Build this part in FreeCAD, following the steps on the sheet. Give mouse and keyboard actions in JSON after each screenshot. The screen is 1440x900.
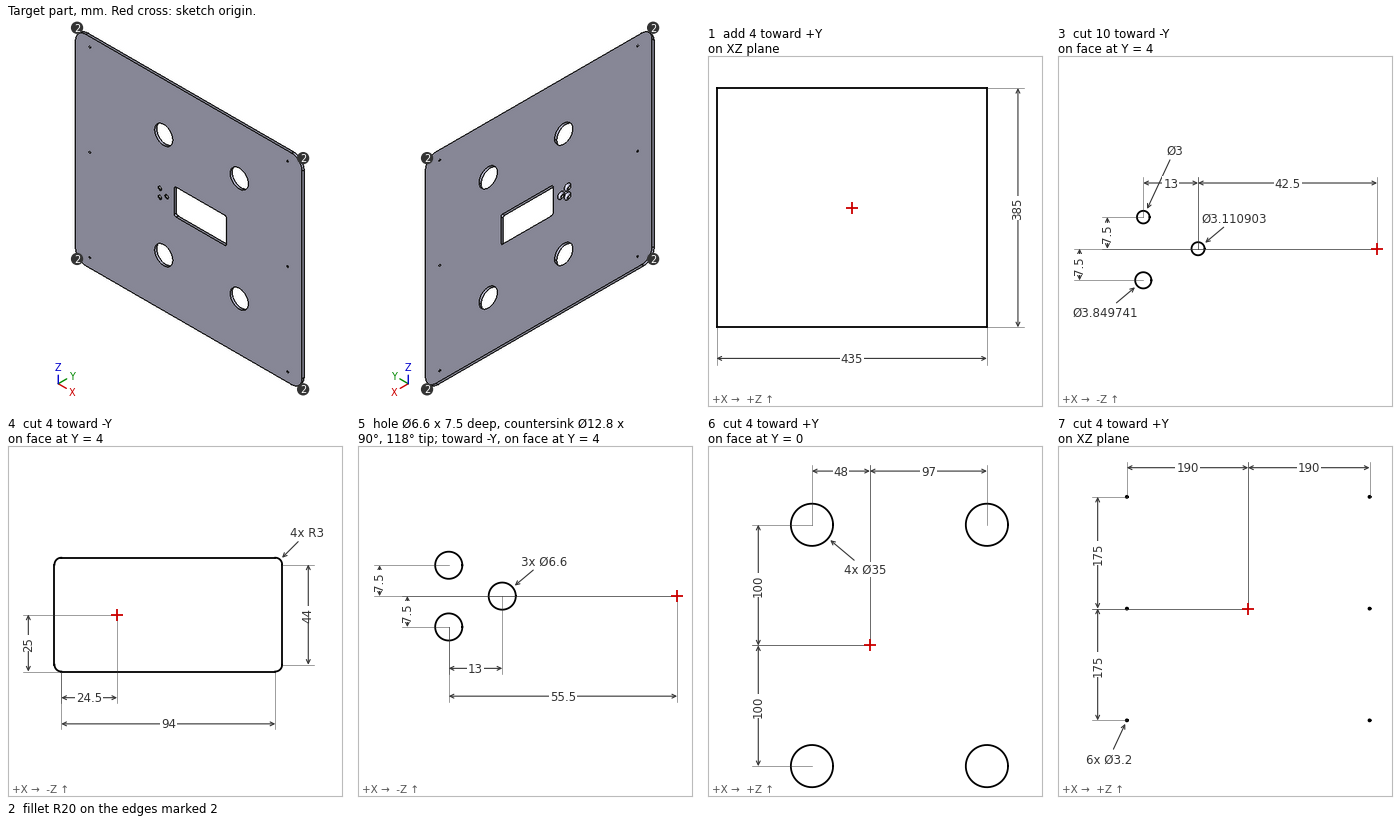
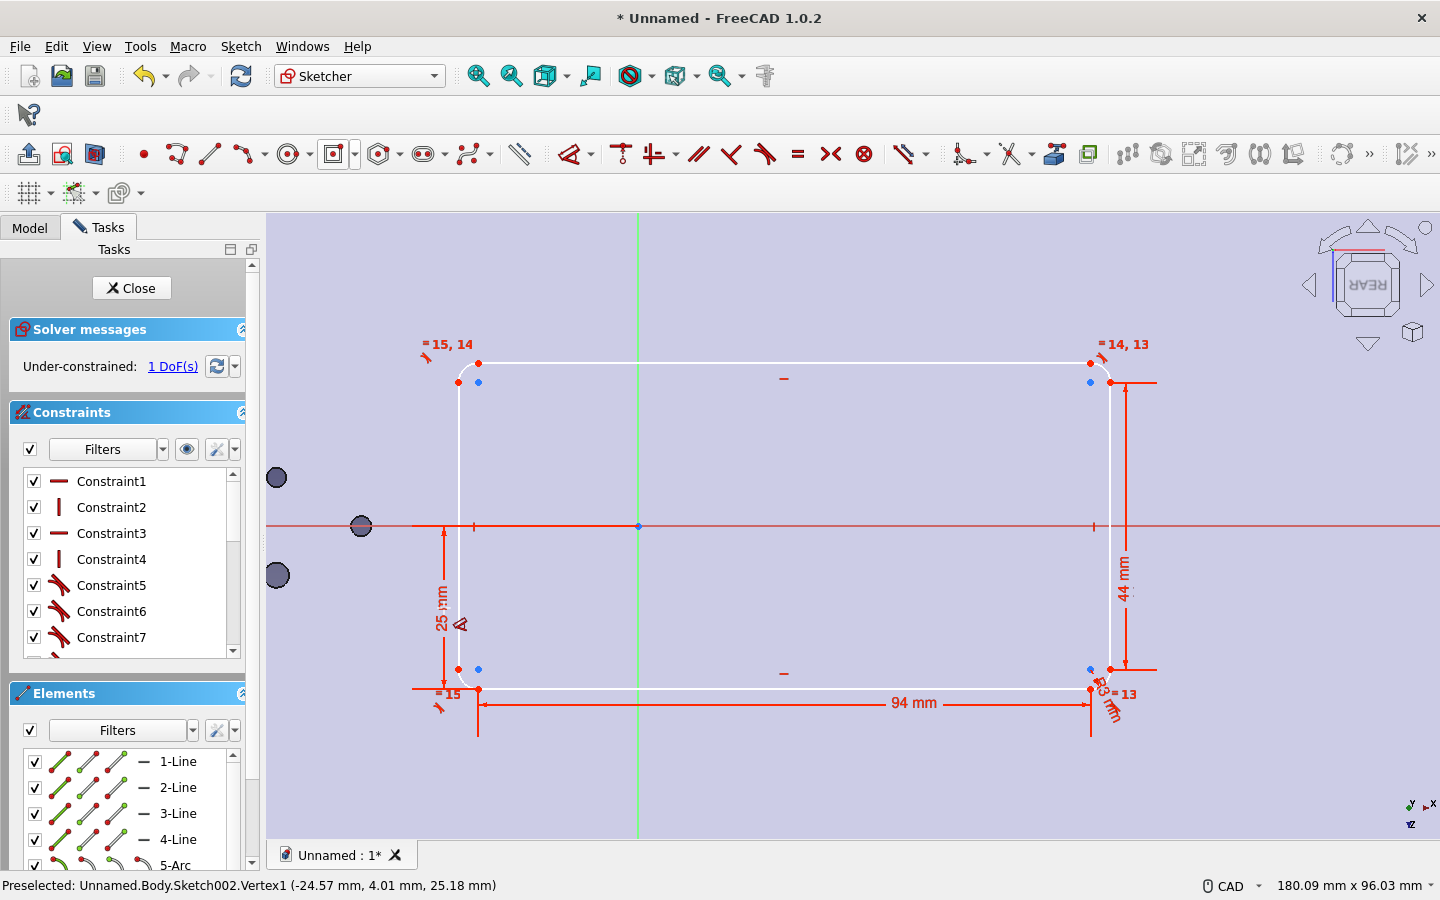
{"action": "left_click", "coordinate": [478, 689]}
{"action": "left_click", "coordinate": [558, 723]}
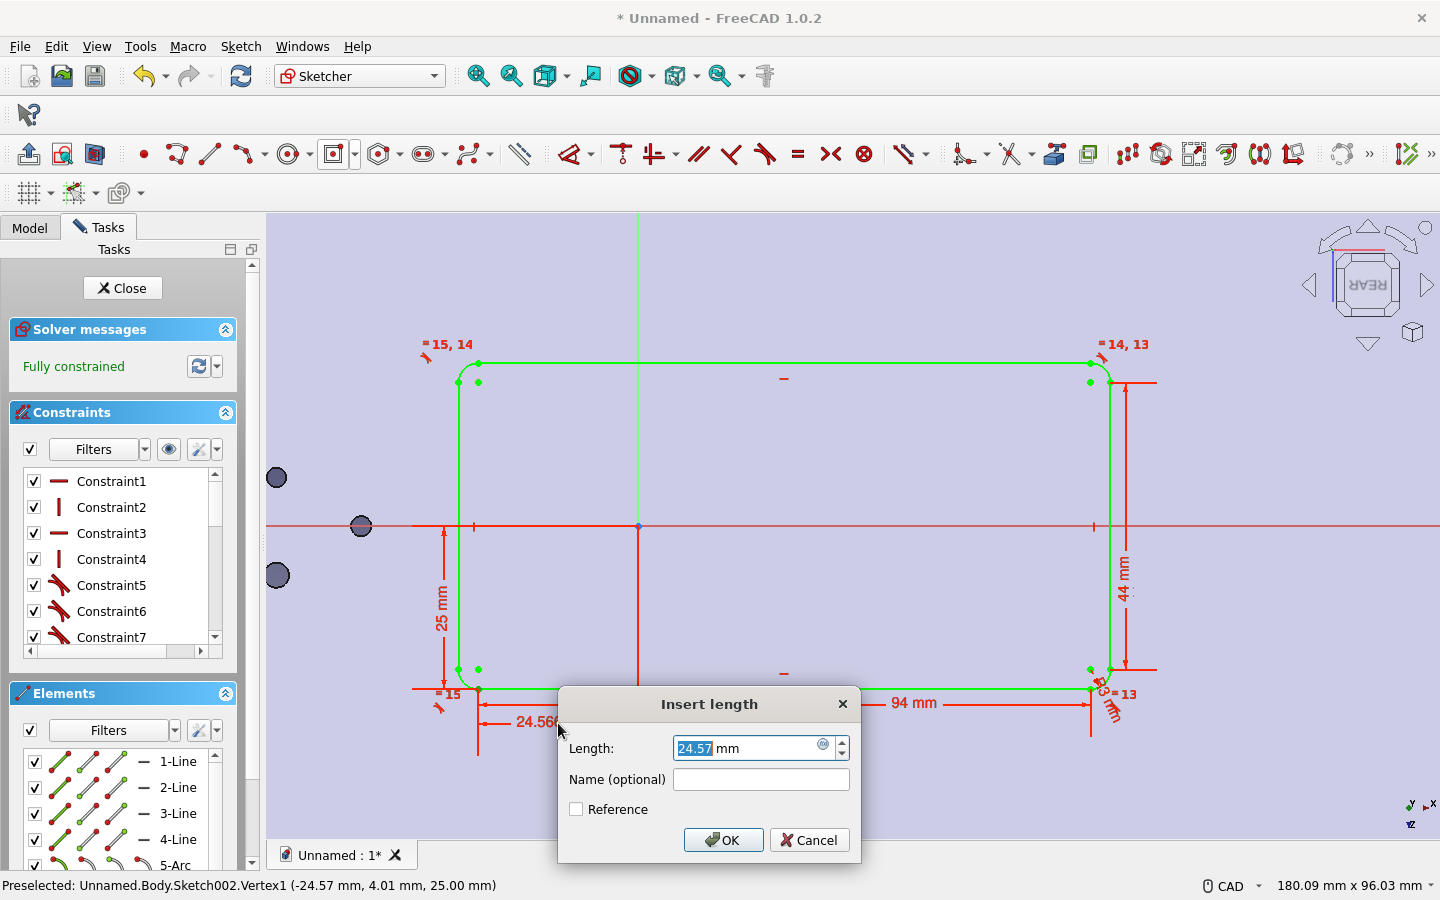
{"action": "type", "text": "24.5"}
{"action": "key", "text": "Return"}
{"action": "key", "text": "Escape"}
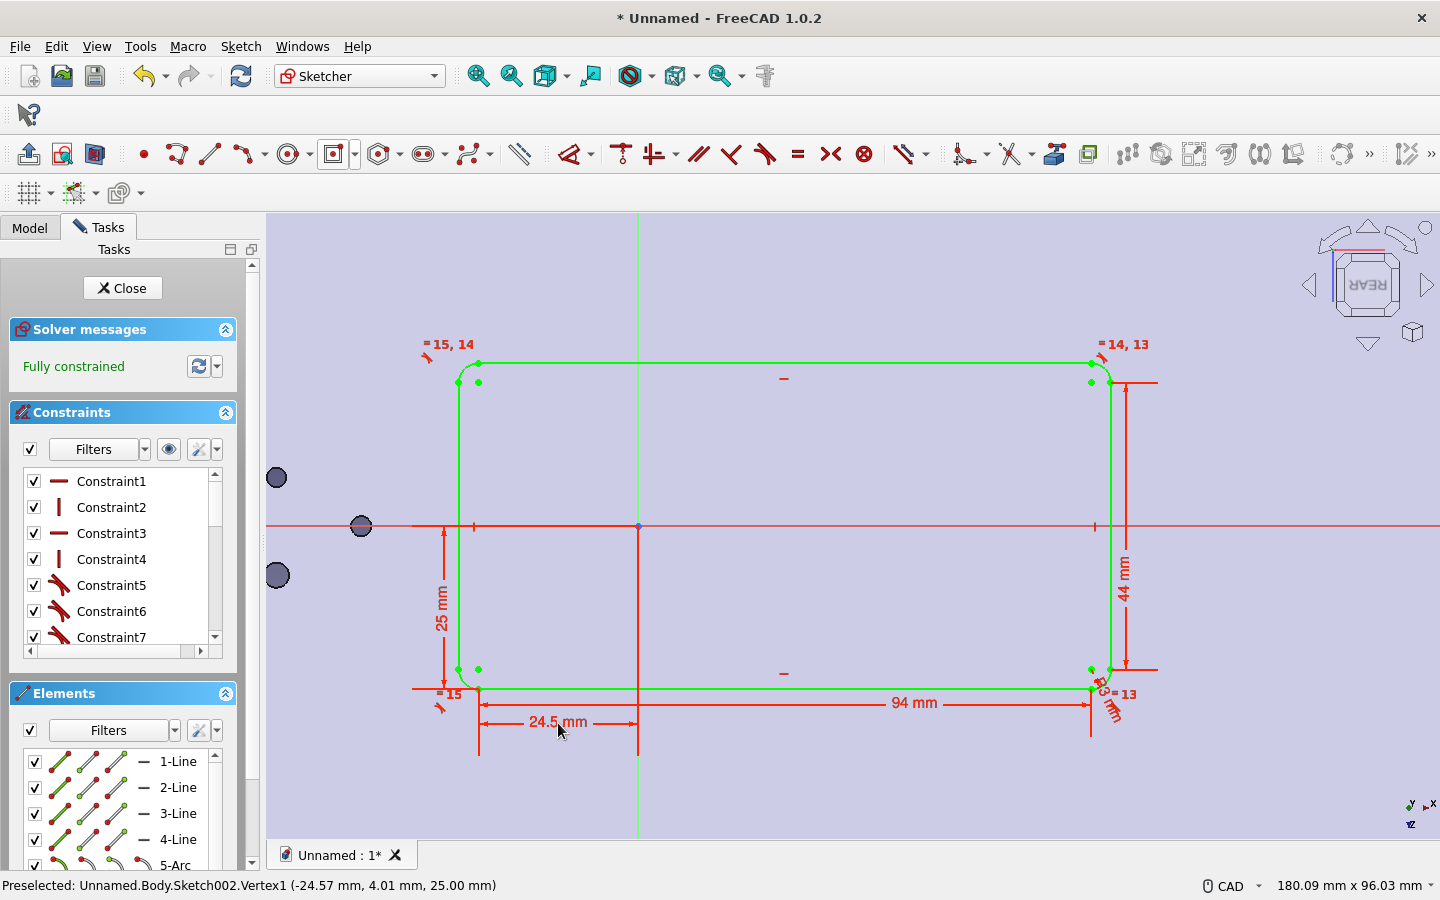
{"action": "left_click", "coordinate": [123, 288]}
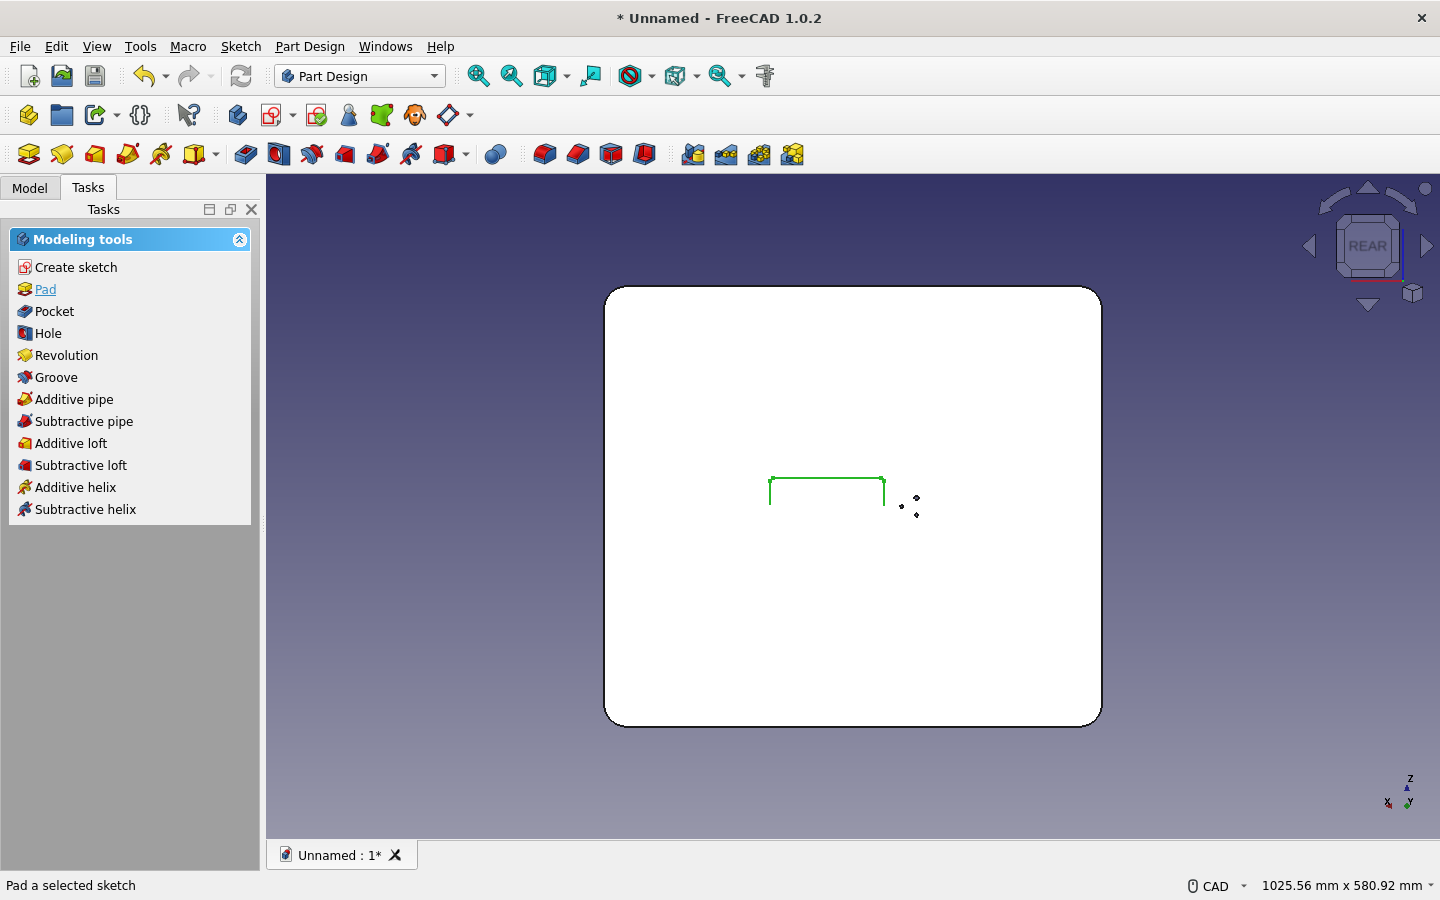
{"action": "left_click", "coordinate": [246, 154]}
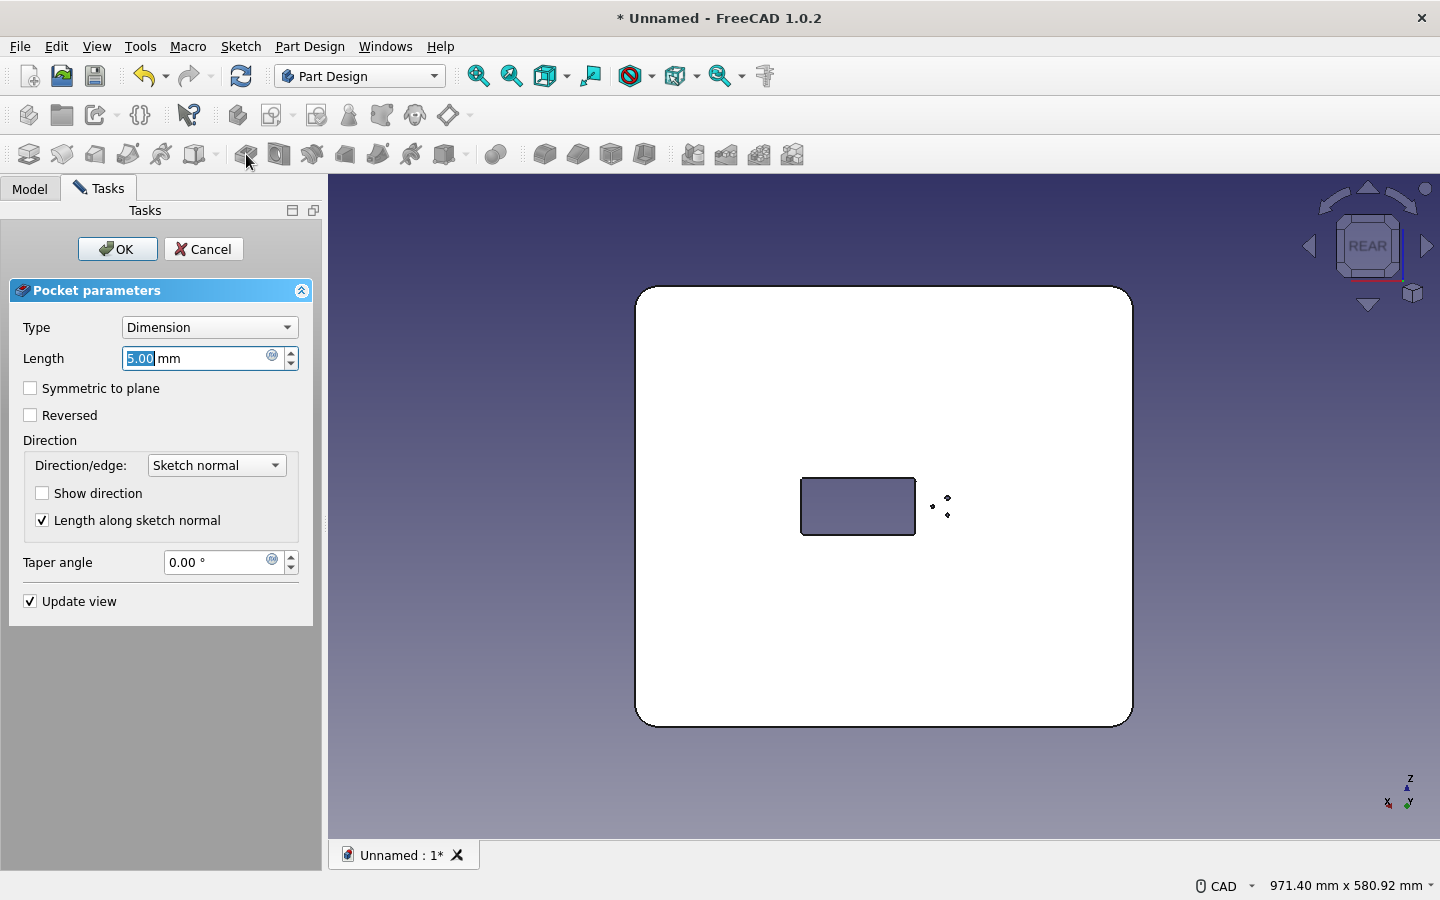
{"action": "type", "text": "4"}
{"action": "key", "text": "Tab"}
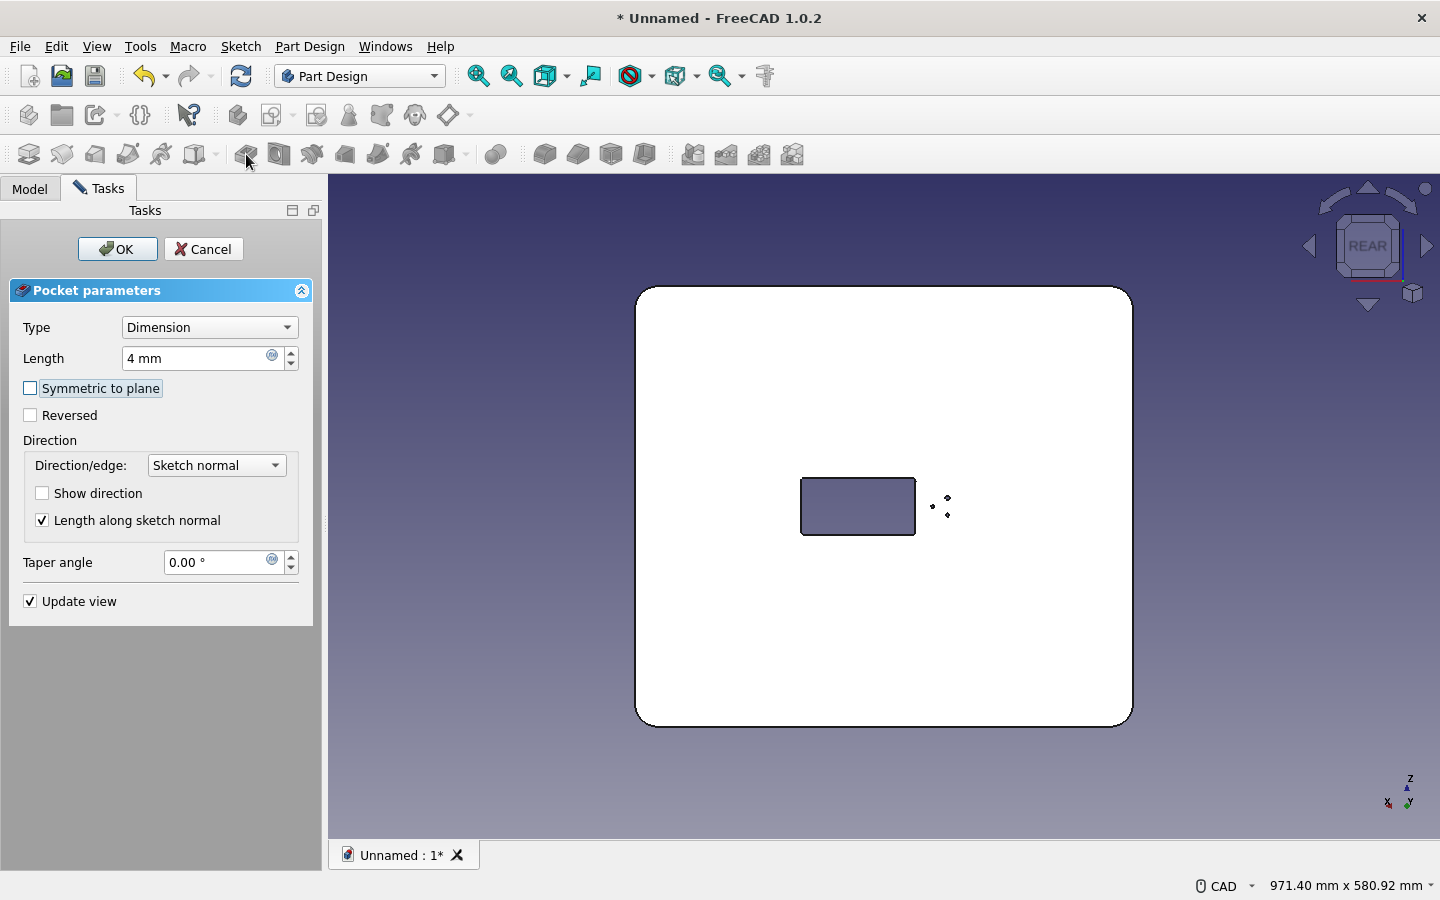
{"action": "left_click", "coordinate": [118, 249]}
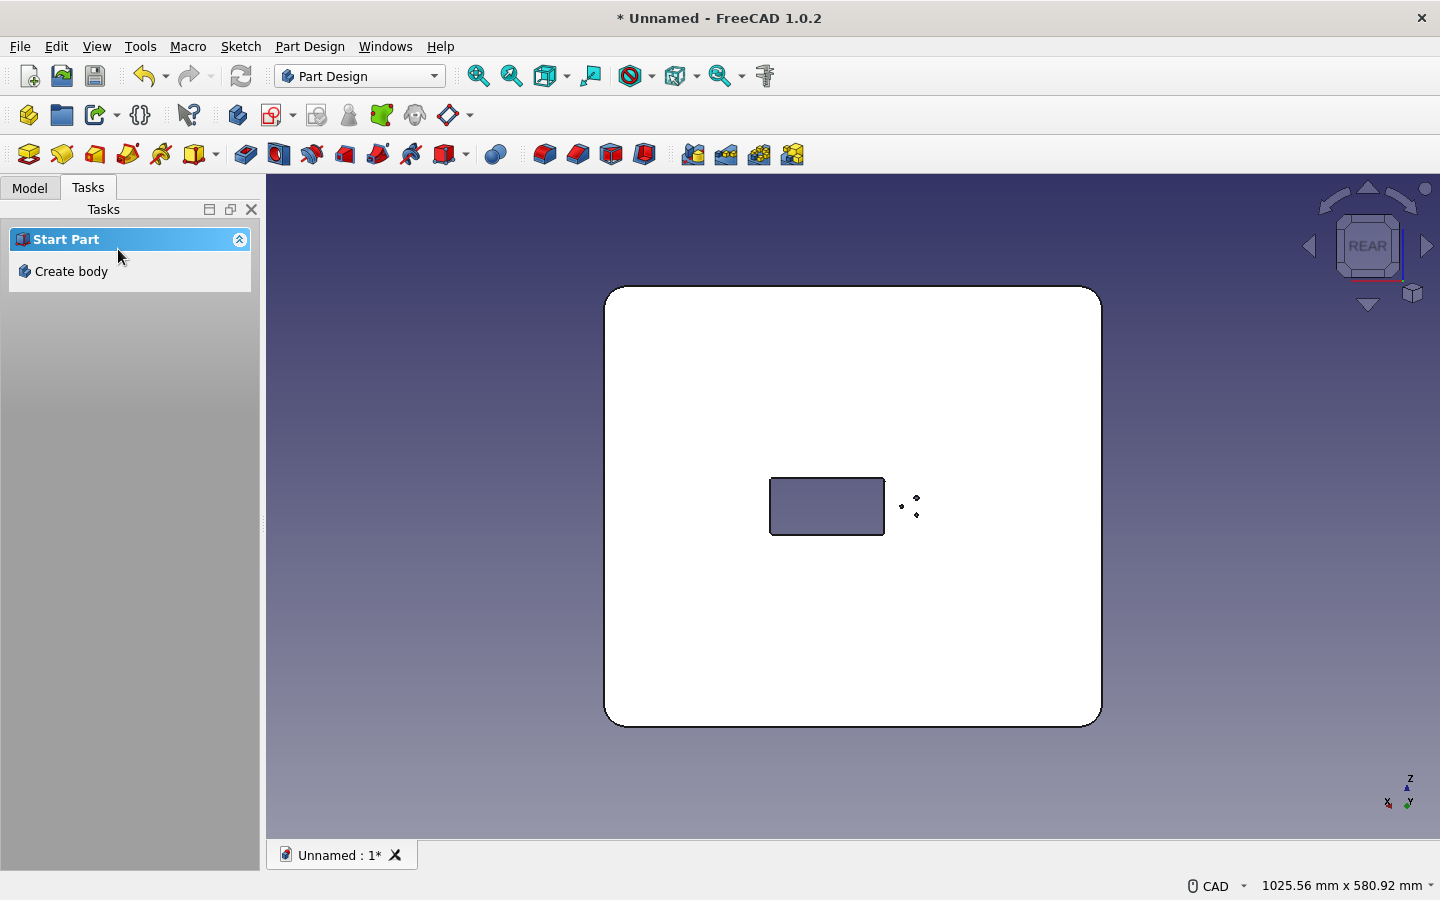
{"action": "left_click", "coordinate": [711, 380]}